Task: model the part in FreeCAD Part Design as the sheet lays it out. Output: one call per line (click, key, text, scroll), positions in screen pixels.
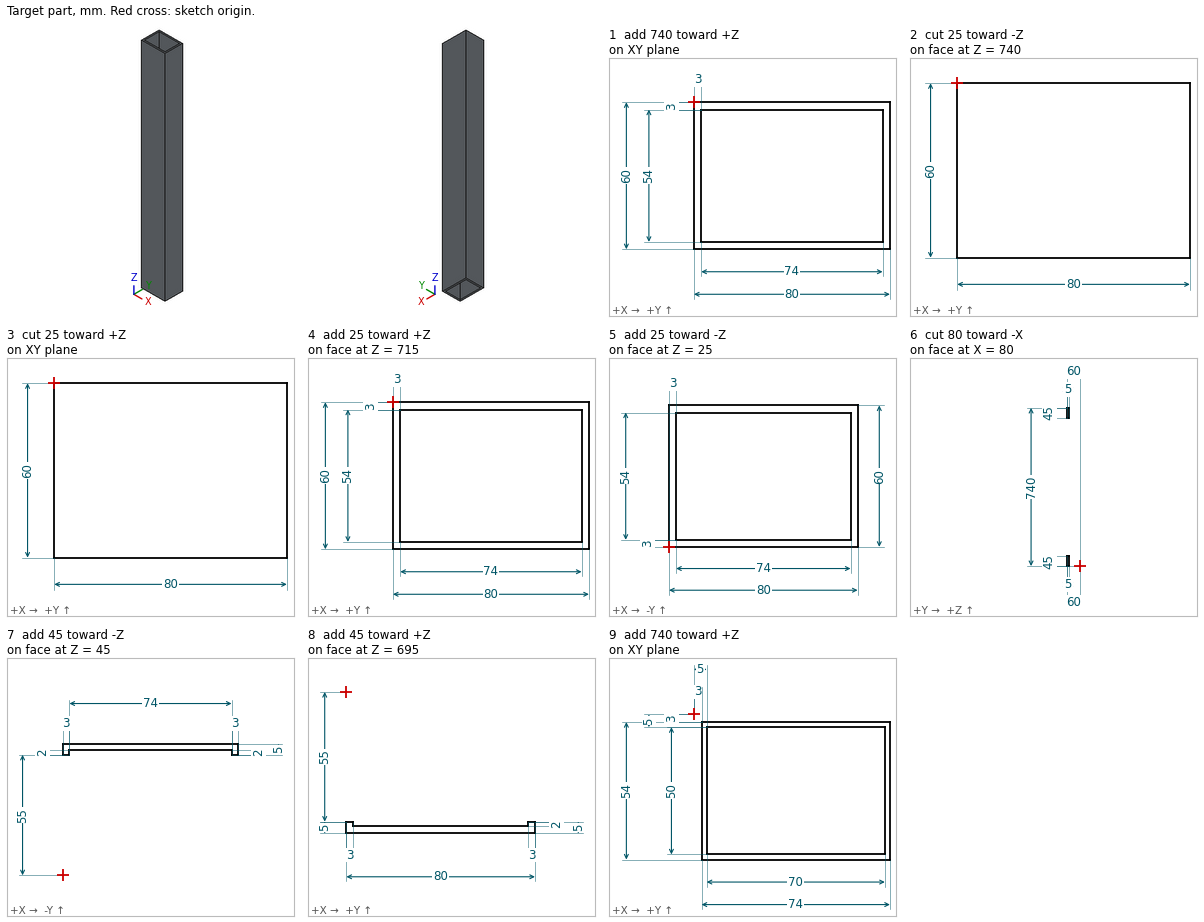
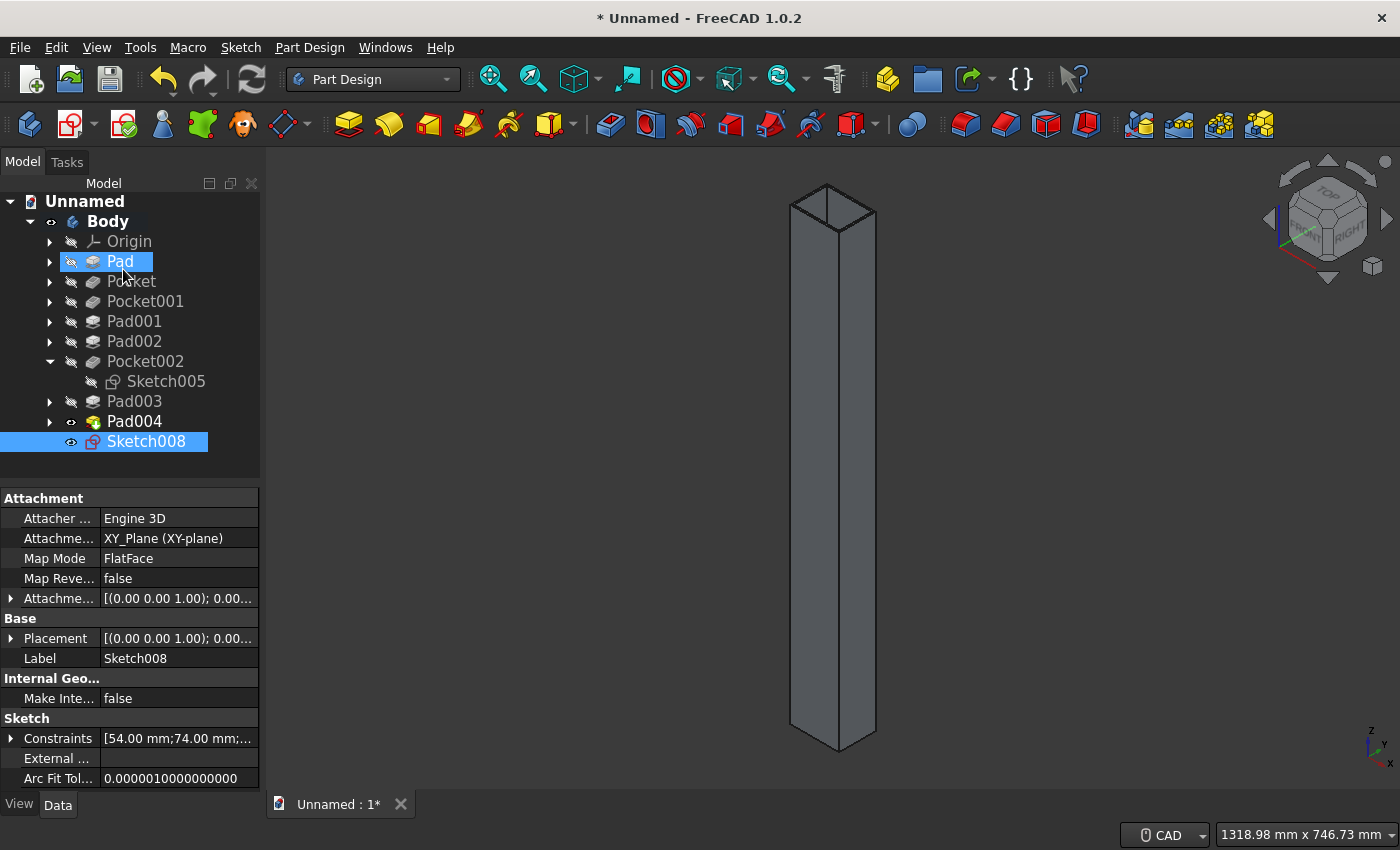
click(350, 124)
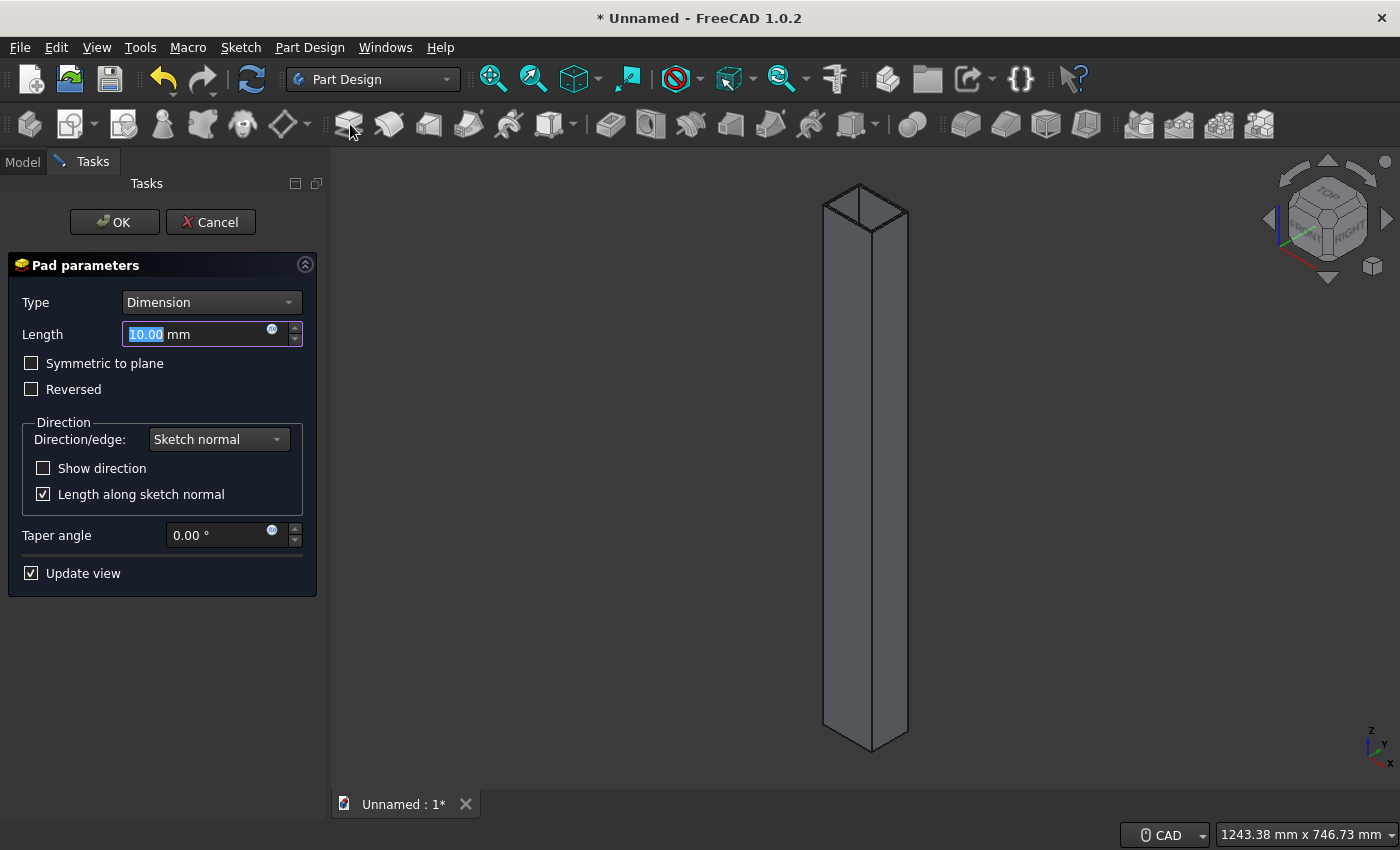
text(740)
key(Tab)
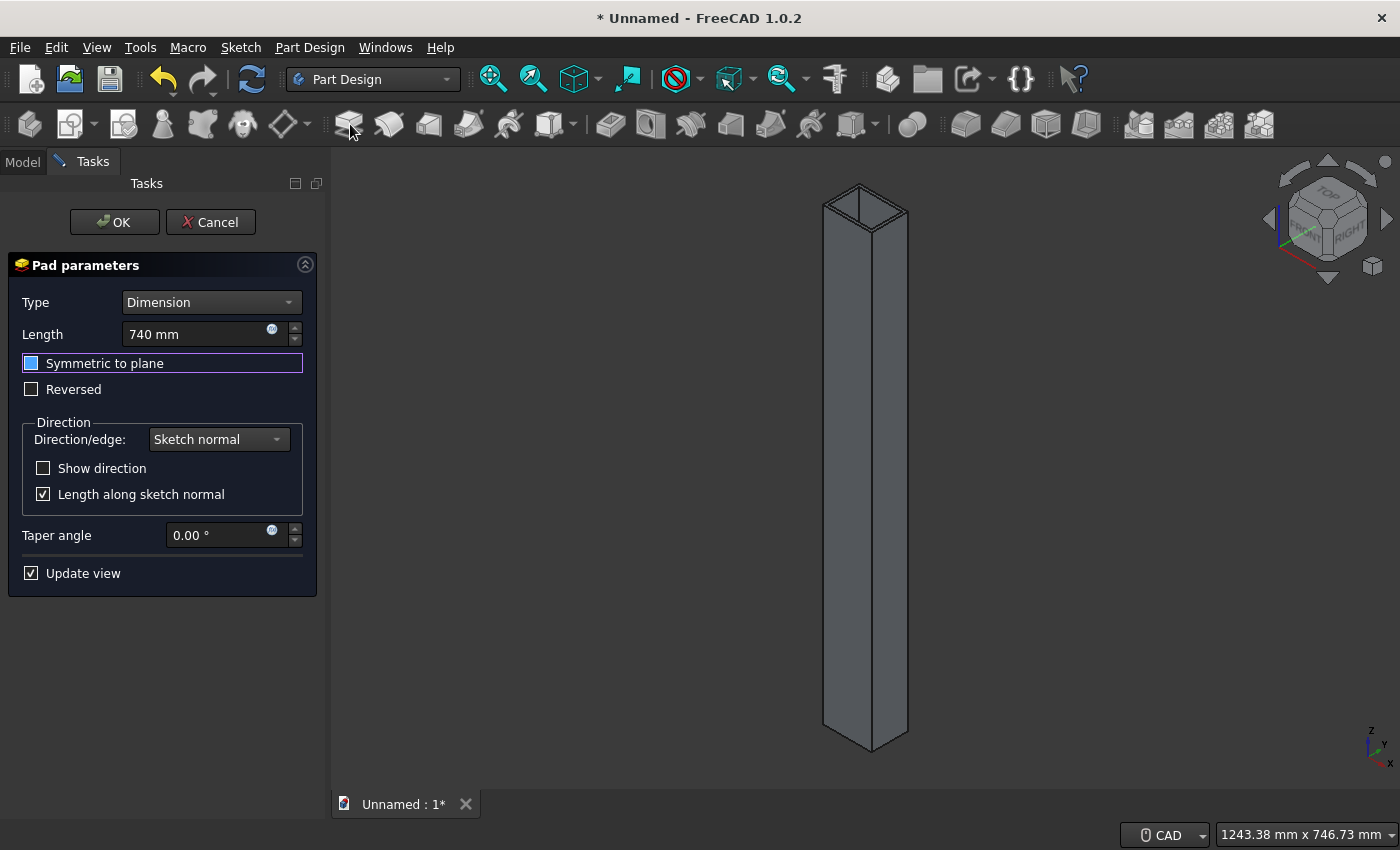
click(115, 222)